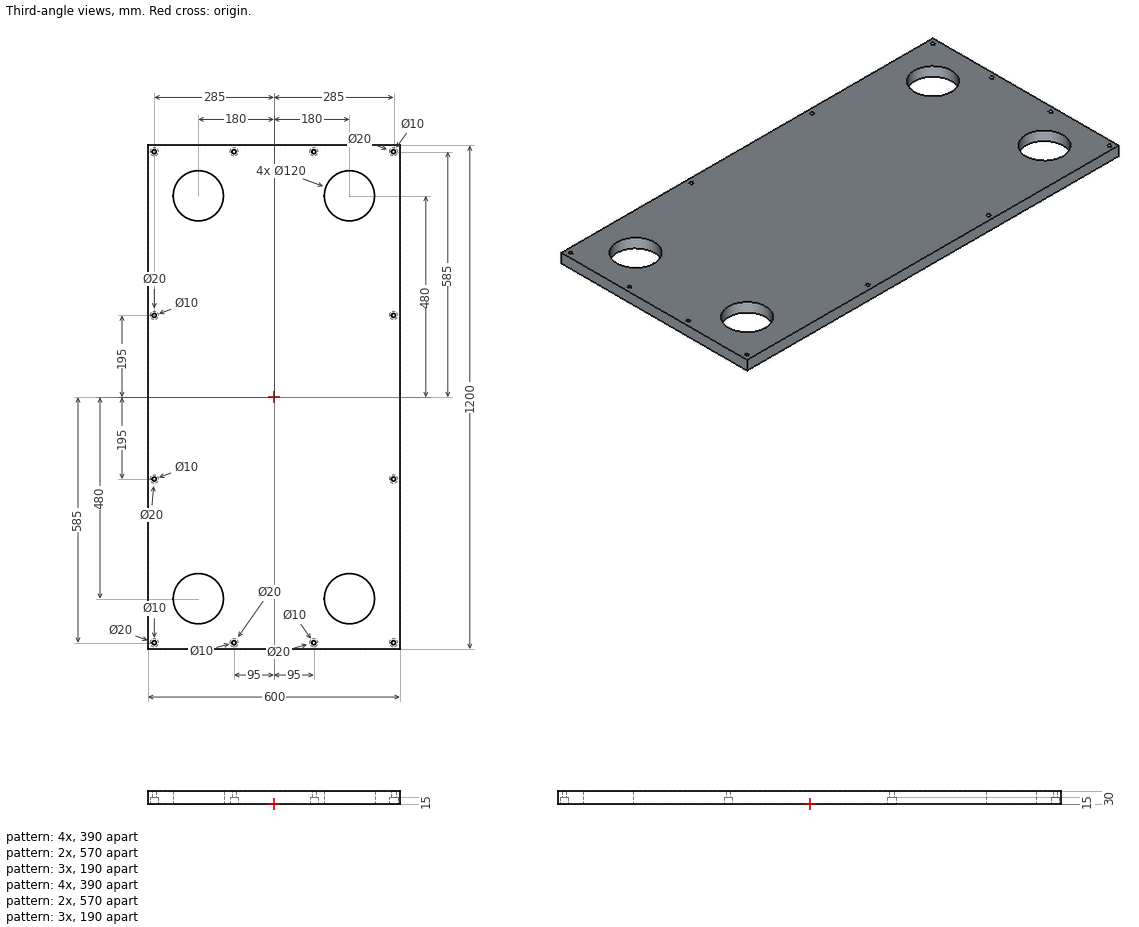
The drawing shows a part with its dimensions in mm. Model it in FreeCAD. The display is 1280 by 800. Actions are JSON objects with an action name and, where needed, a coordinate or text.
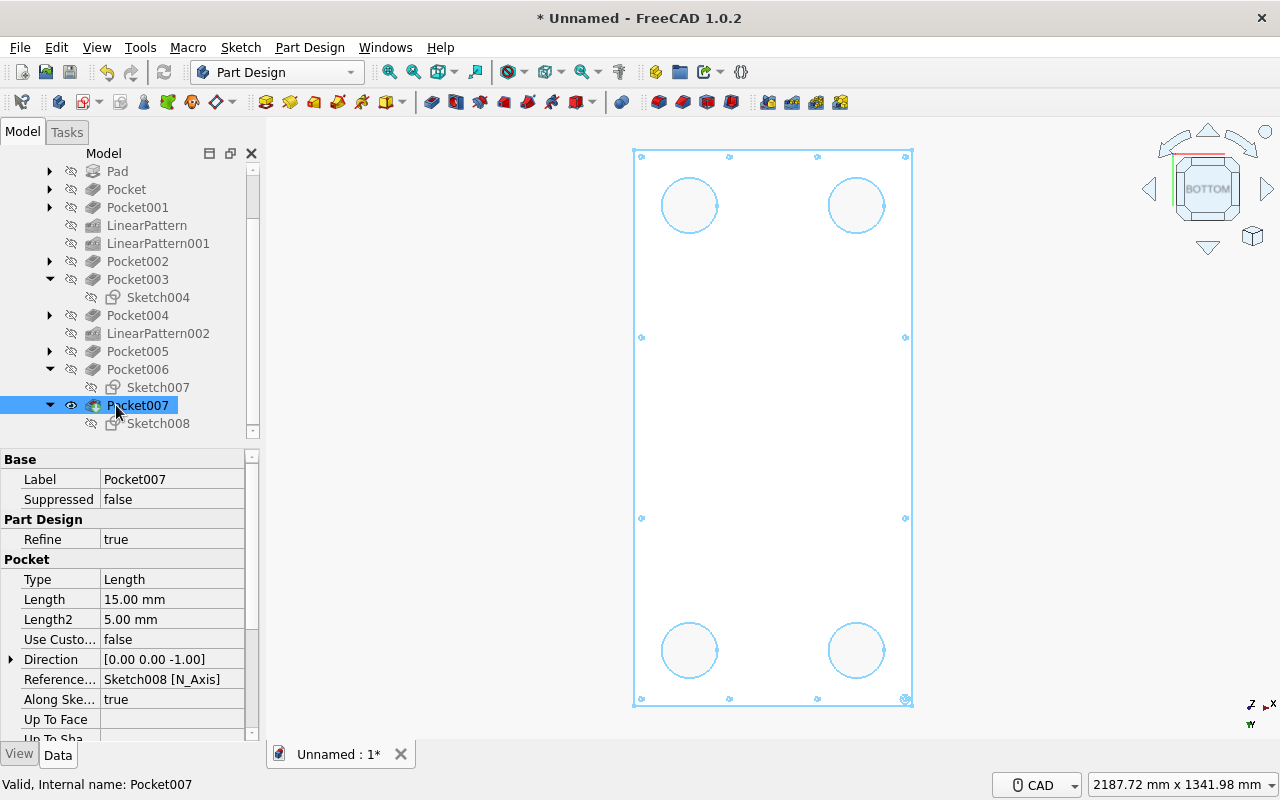
{"action": "left_click", "coordinate": [792, 102]}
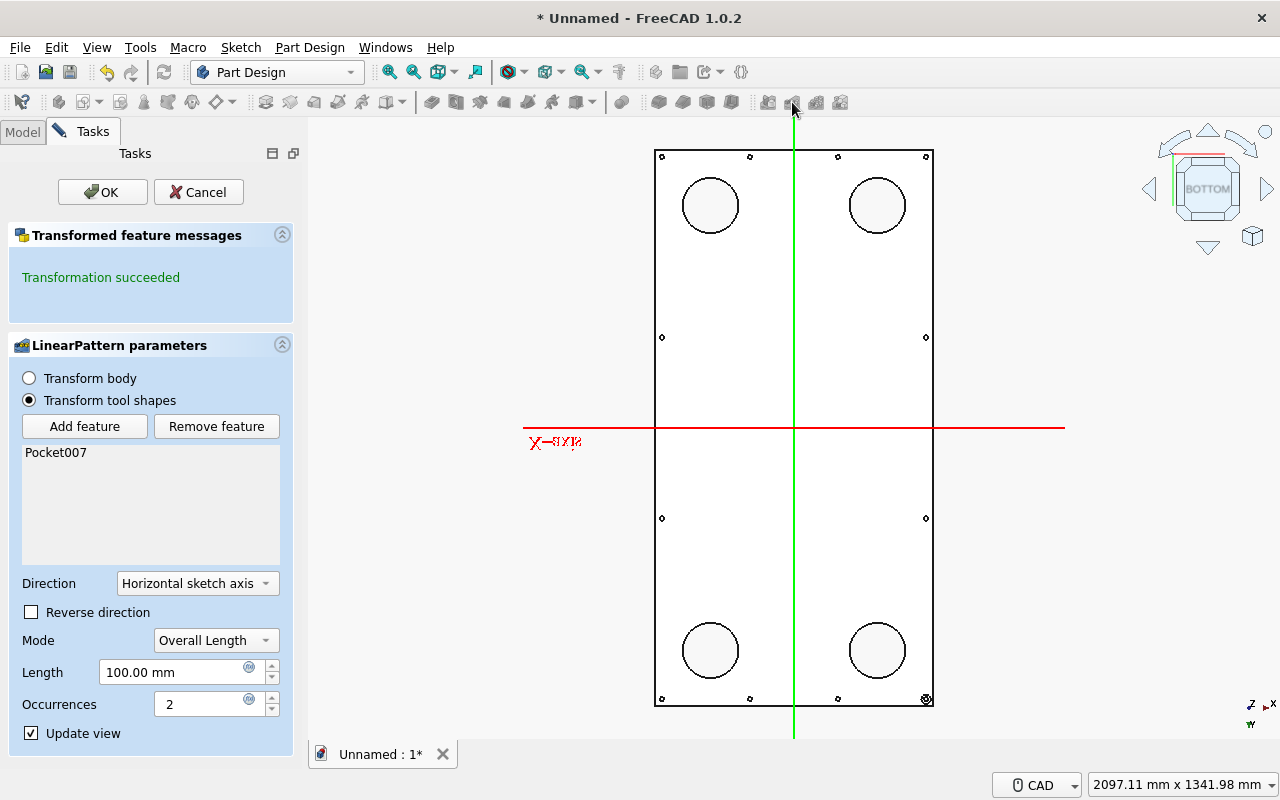
{"action": "left_click", "coordinate": [198, 584]}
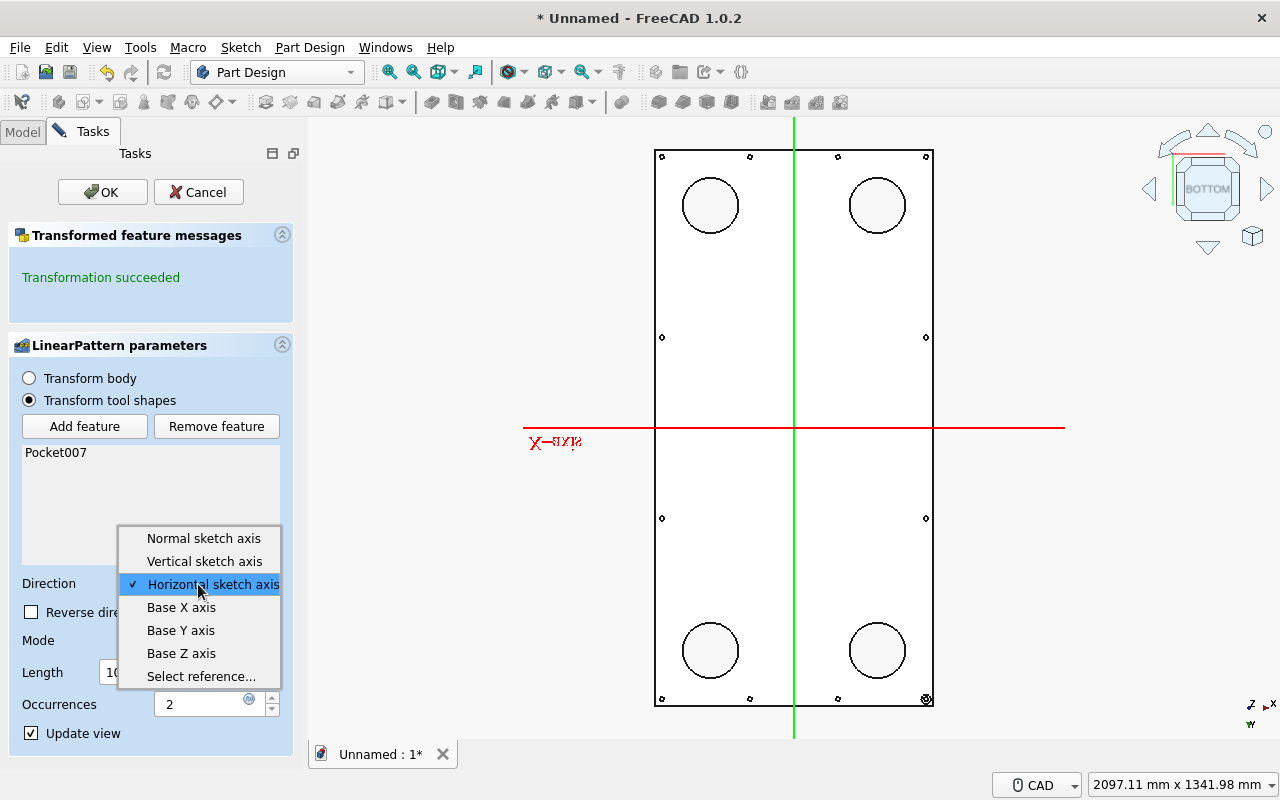
{"action": "left_click", "coordinate": [198, 630]}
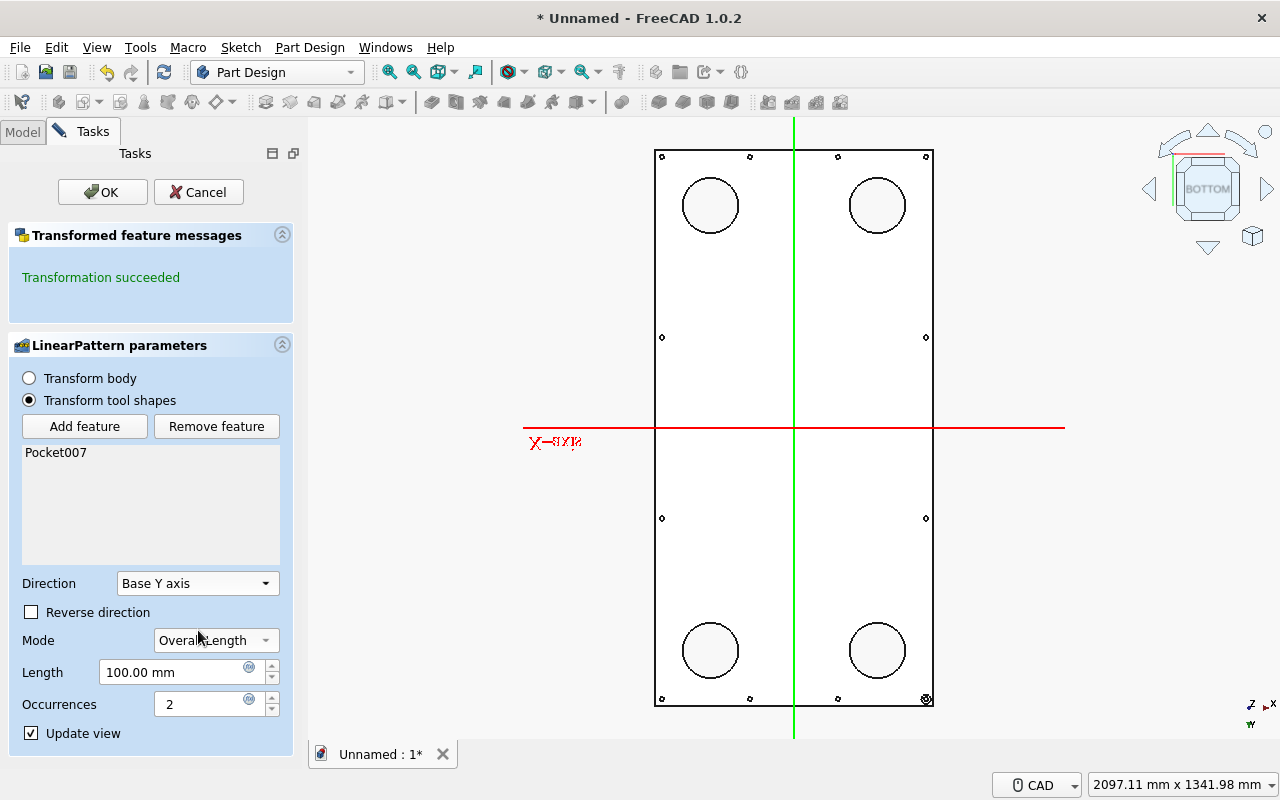
{"action": "left_click", "coordinate": [217, 640]}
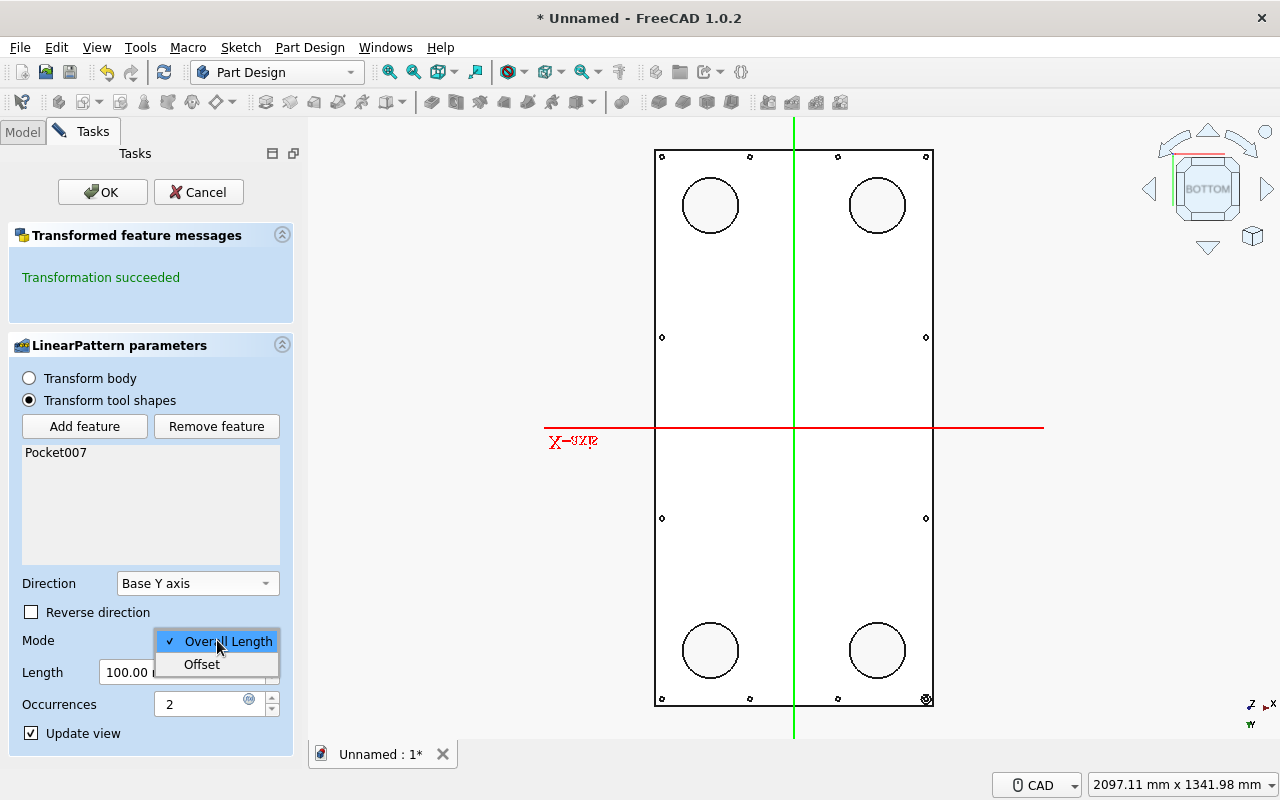
{"action": "left_click", "coordinate": [216, 664]}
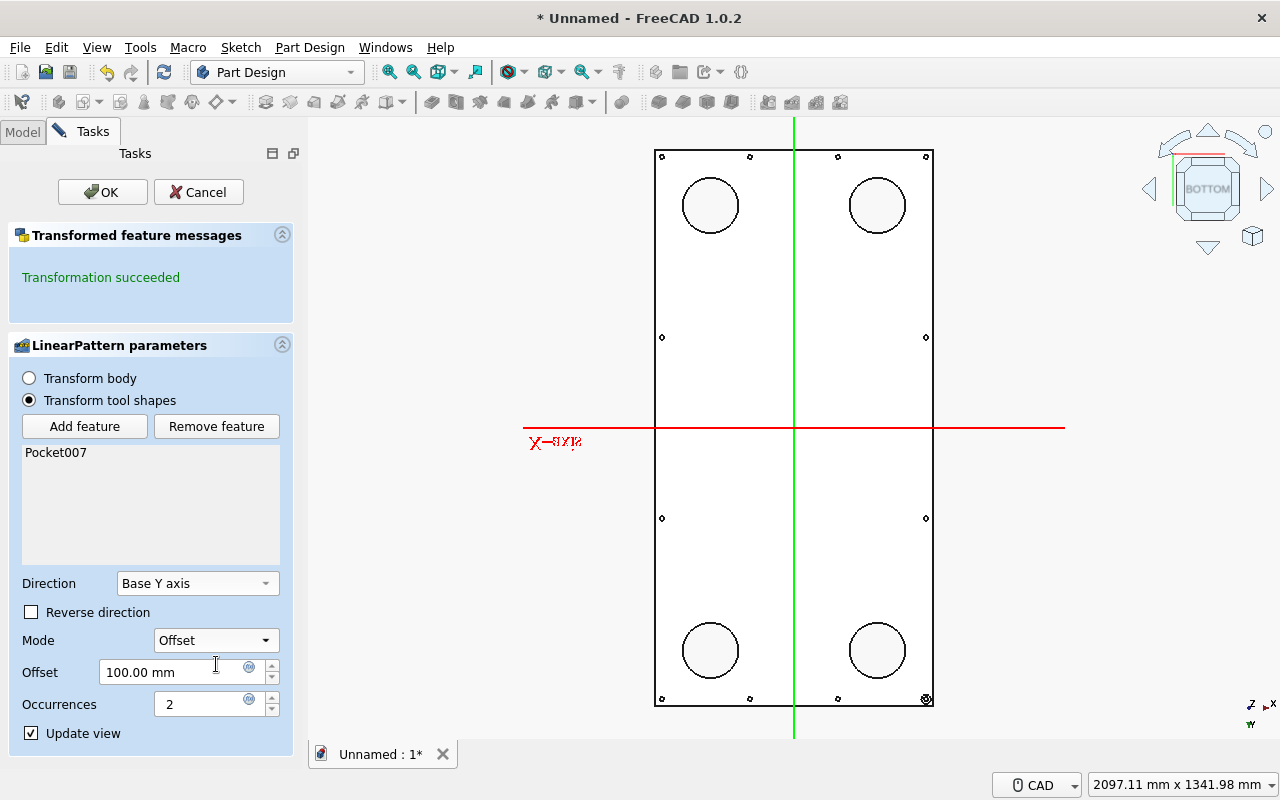
{"action": "triple_click", "coordinate": [182, 672]}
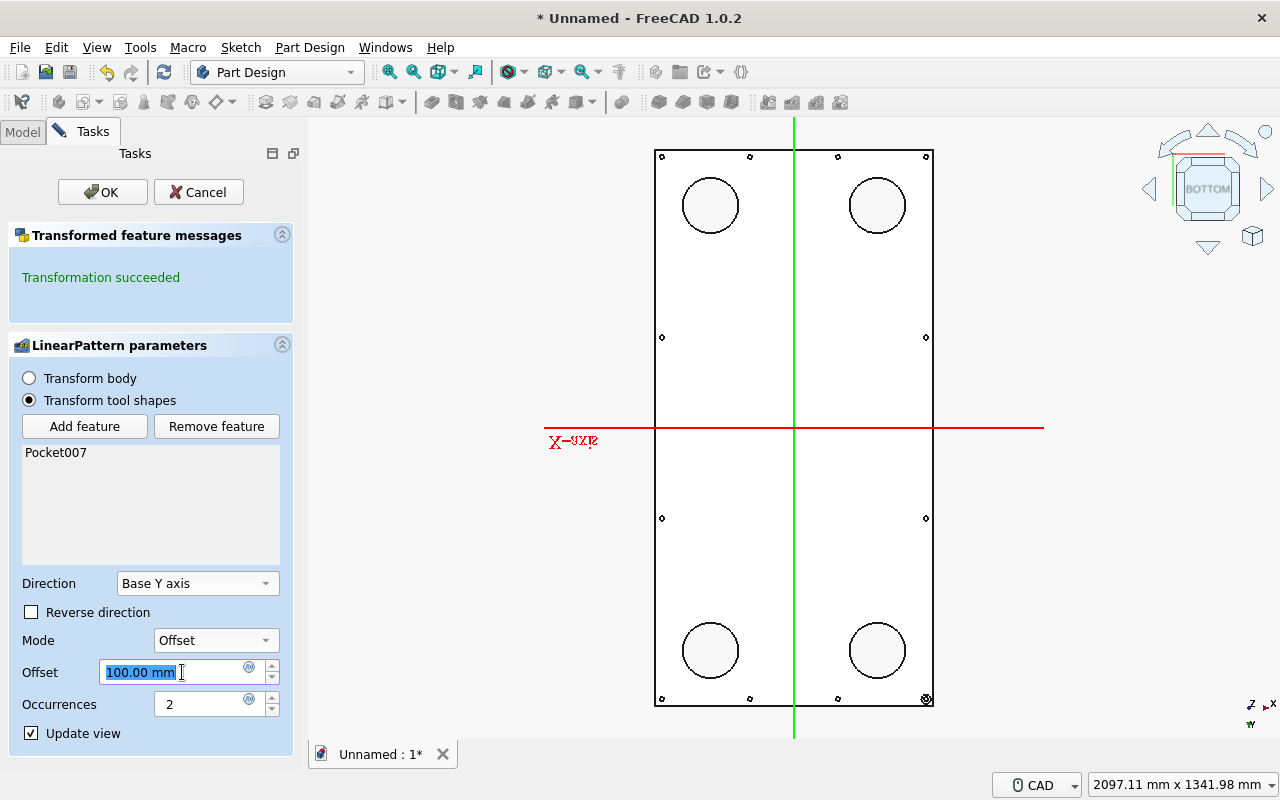
{"action": "type", "text": "390"}
{"action": "key", "text": "Tab"}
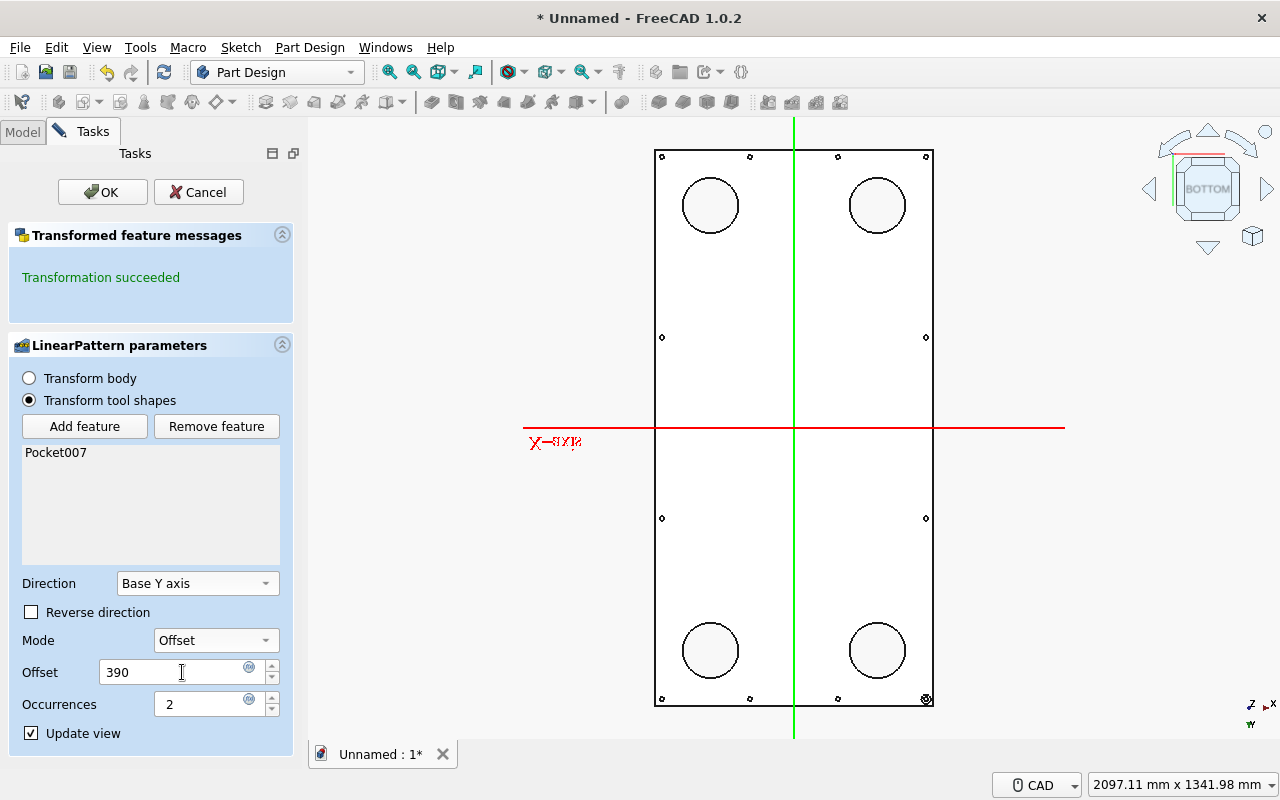
{"action": "triple_click", "coordinate": [209, 704]}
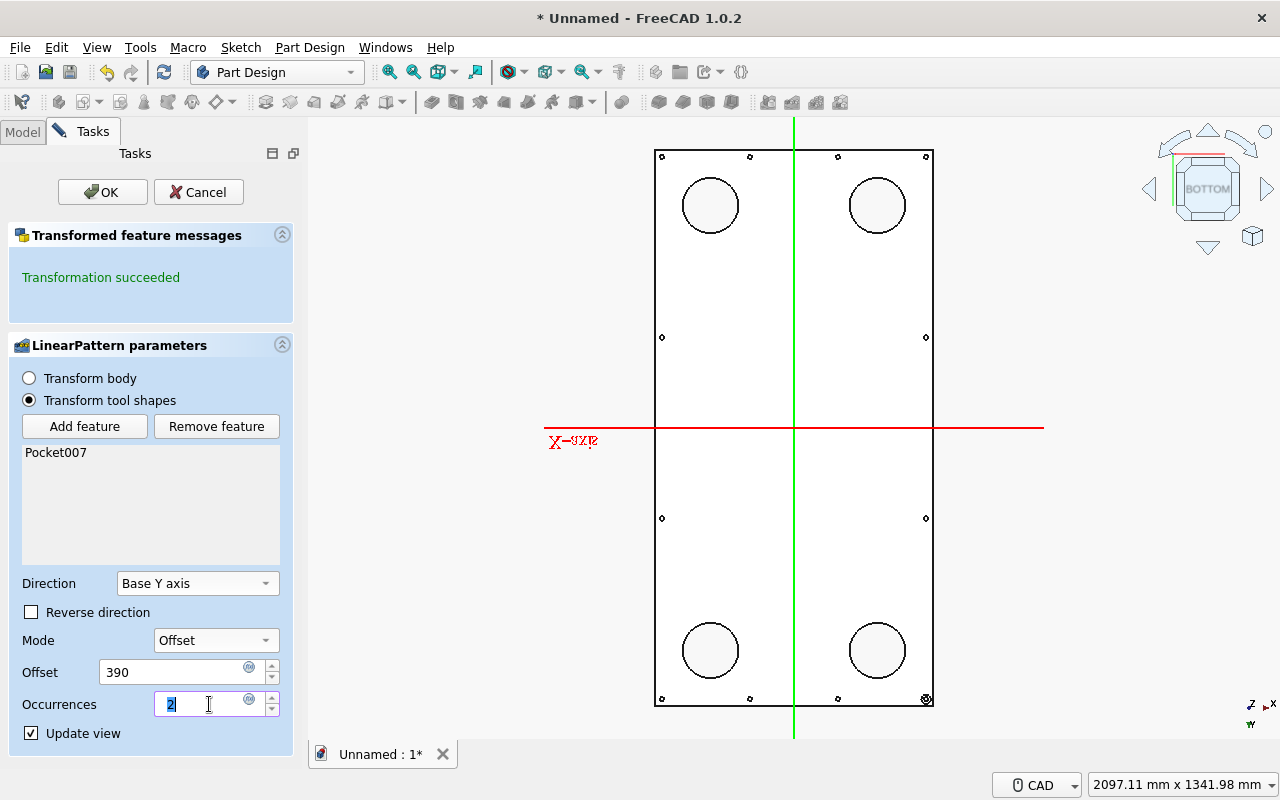
{"action": "type", "text": "4"}
{"action": "key", "text": "Tab"}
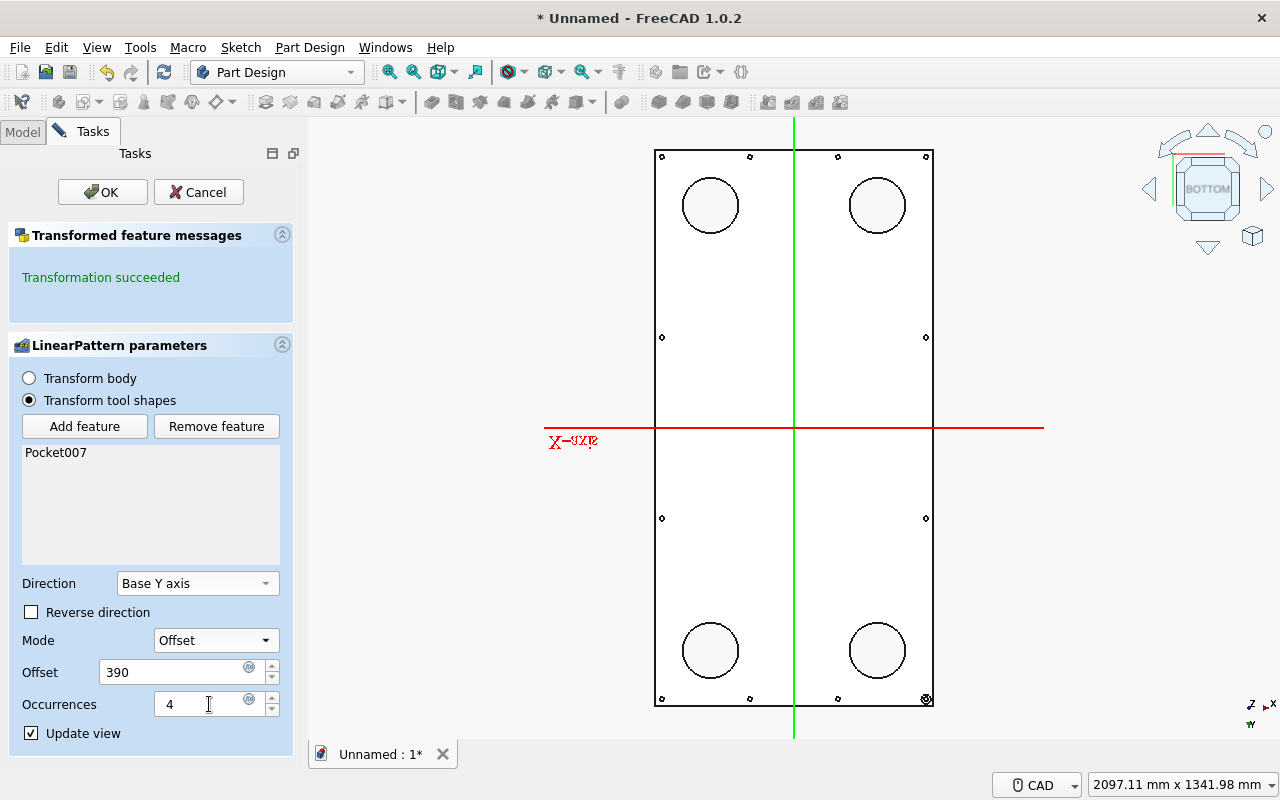
{"action": "left_click", "coordinate": [30, 612]}